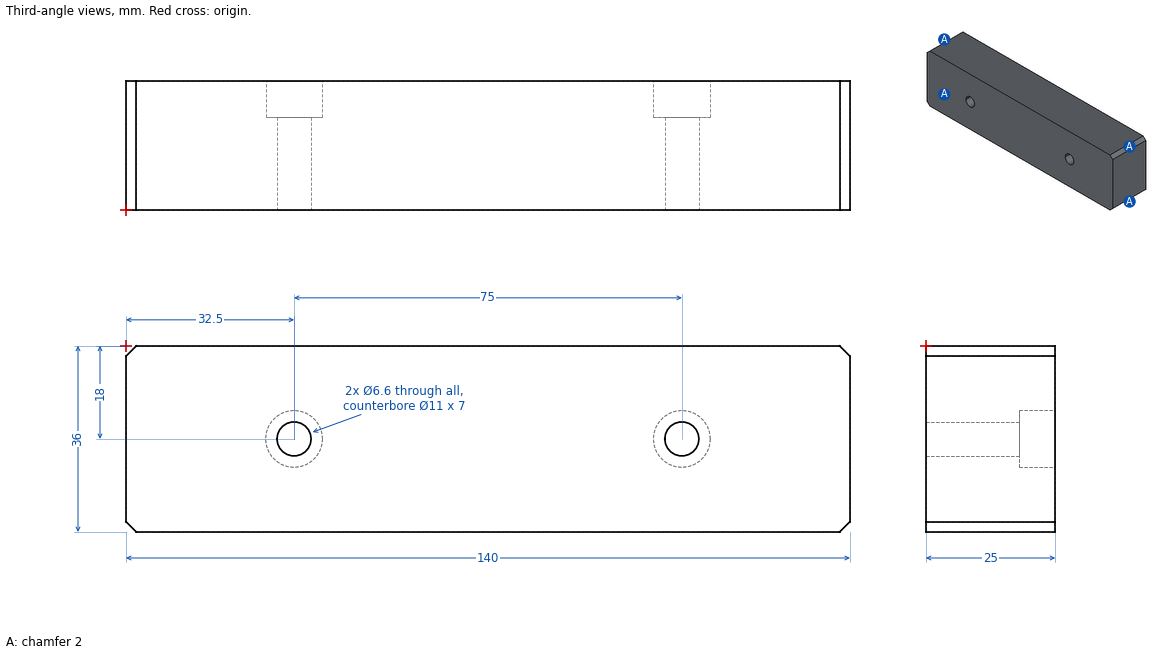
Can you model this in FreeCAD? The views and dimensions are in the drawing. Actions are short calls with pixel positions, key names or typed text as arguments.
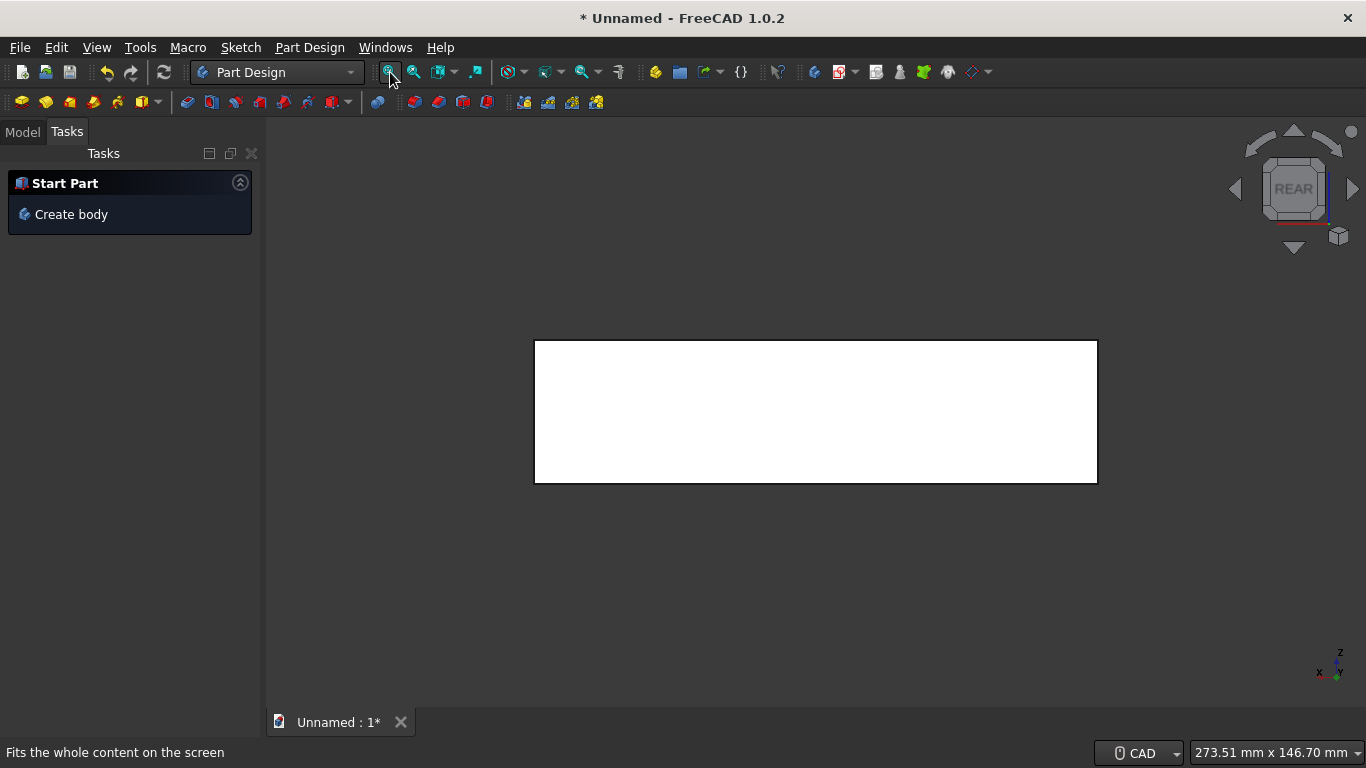
click(655, 411)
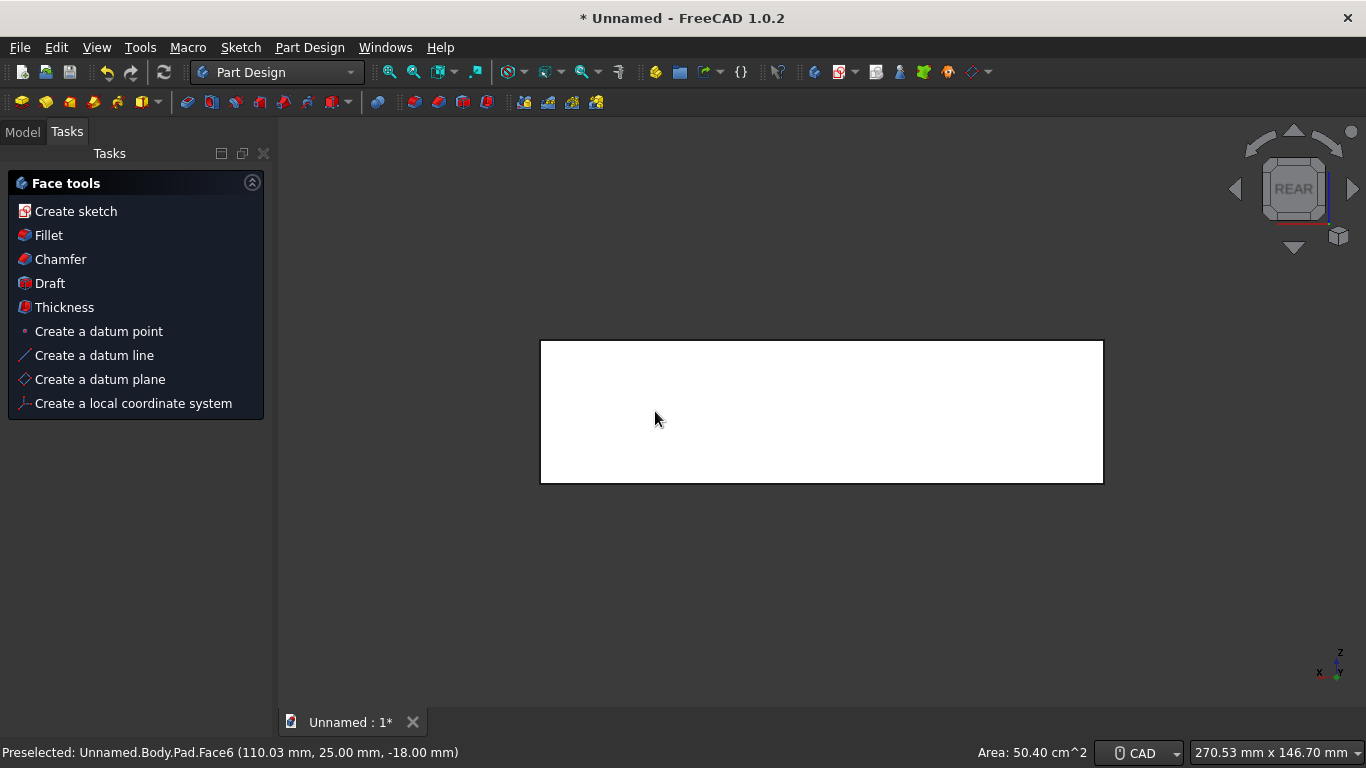
click(840, 72)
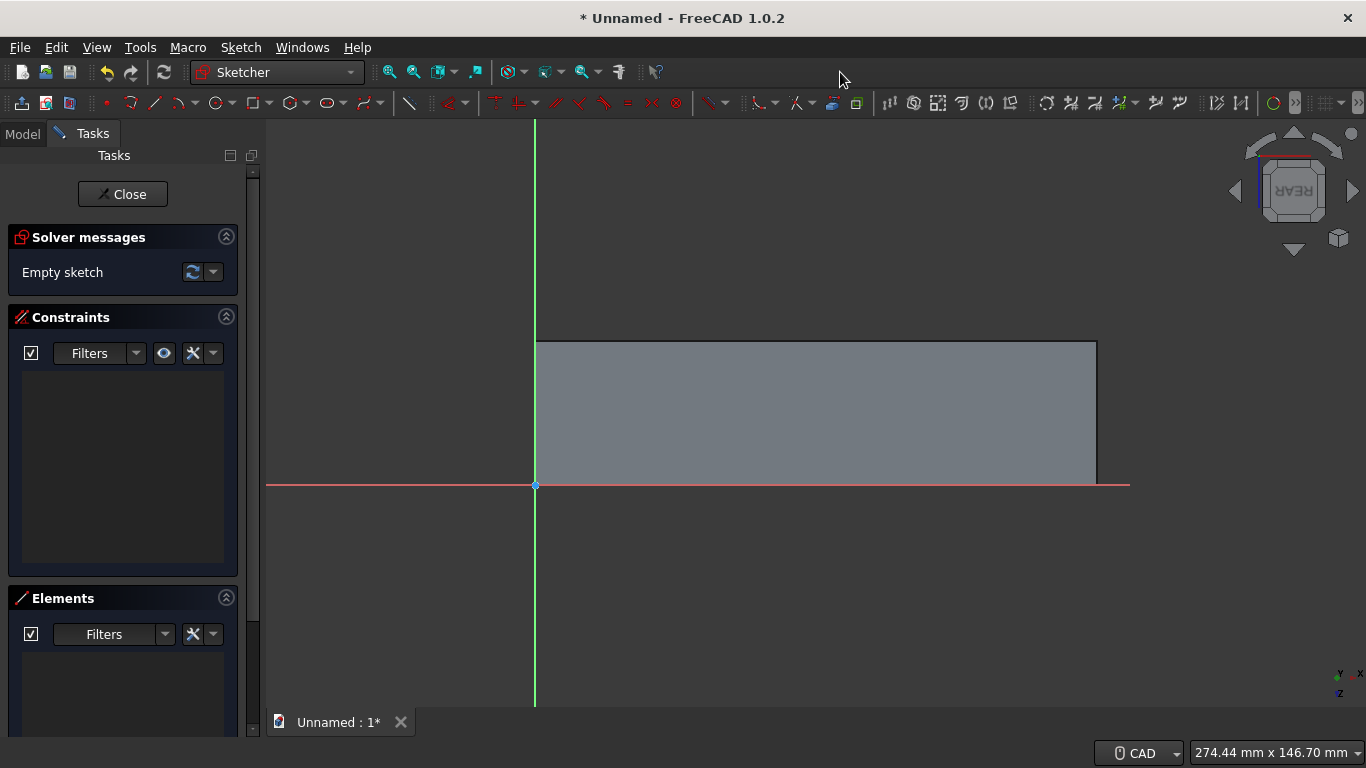
scroll(778, 502, up, 2)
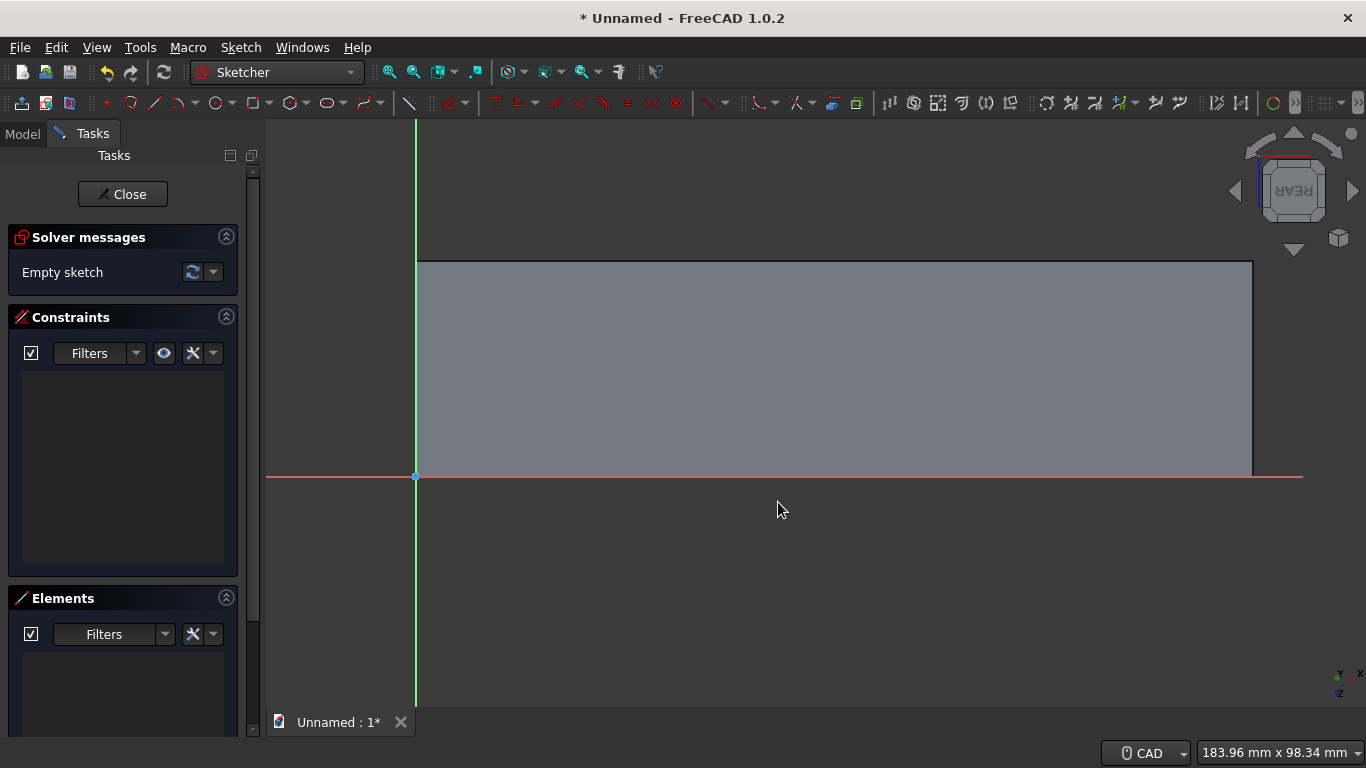
click(216, 104)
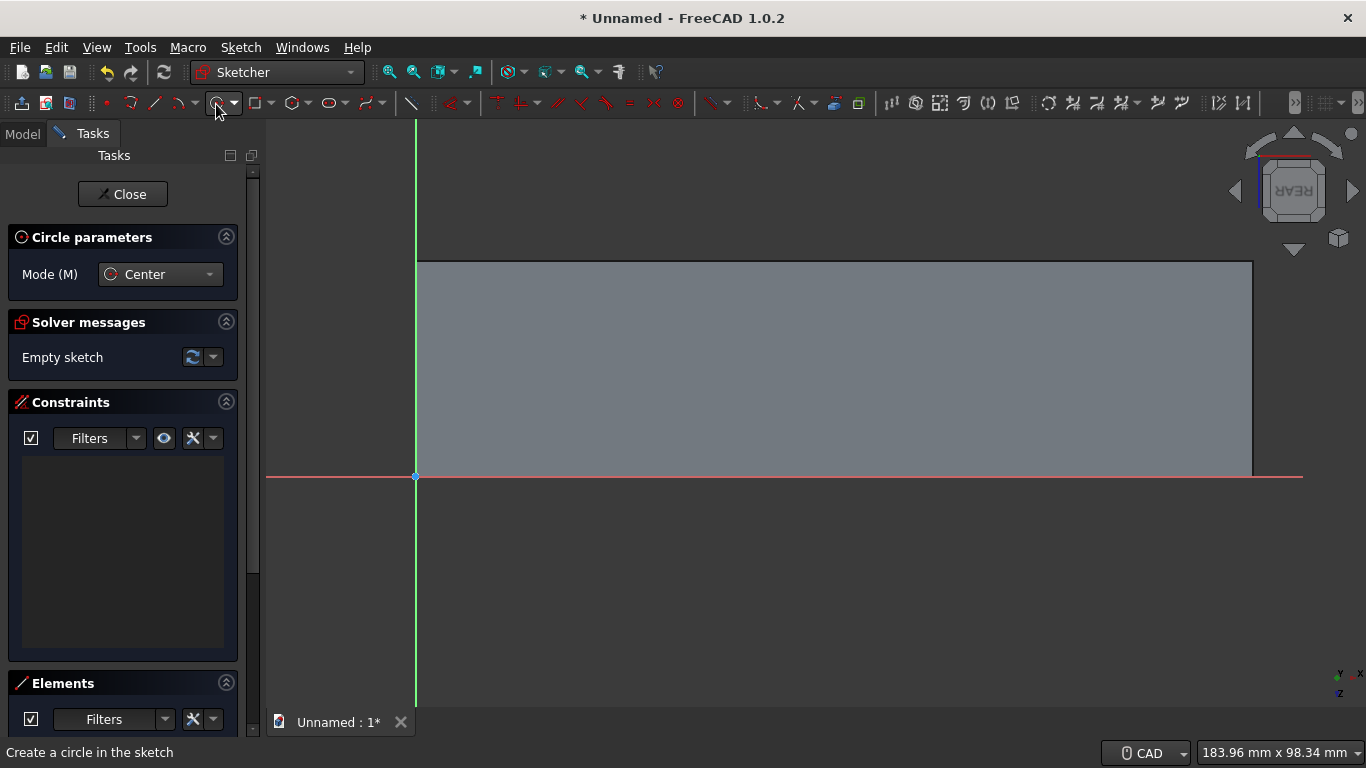
click(610, 369)
click(624, 355)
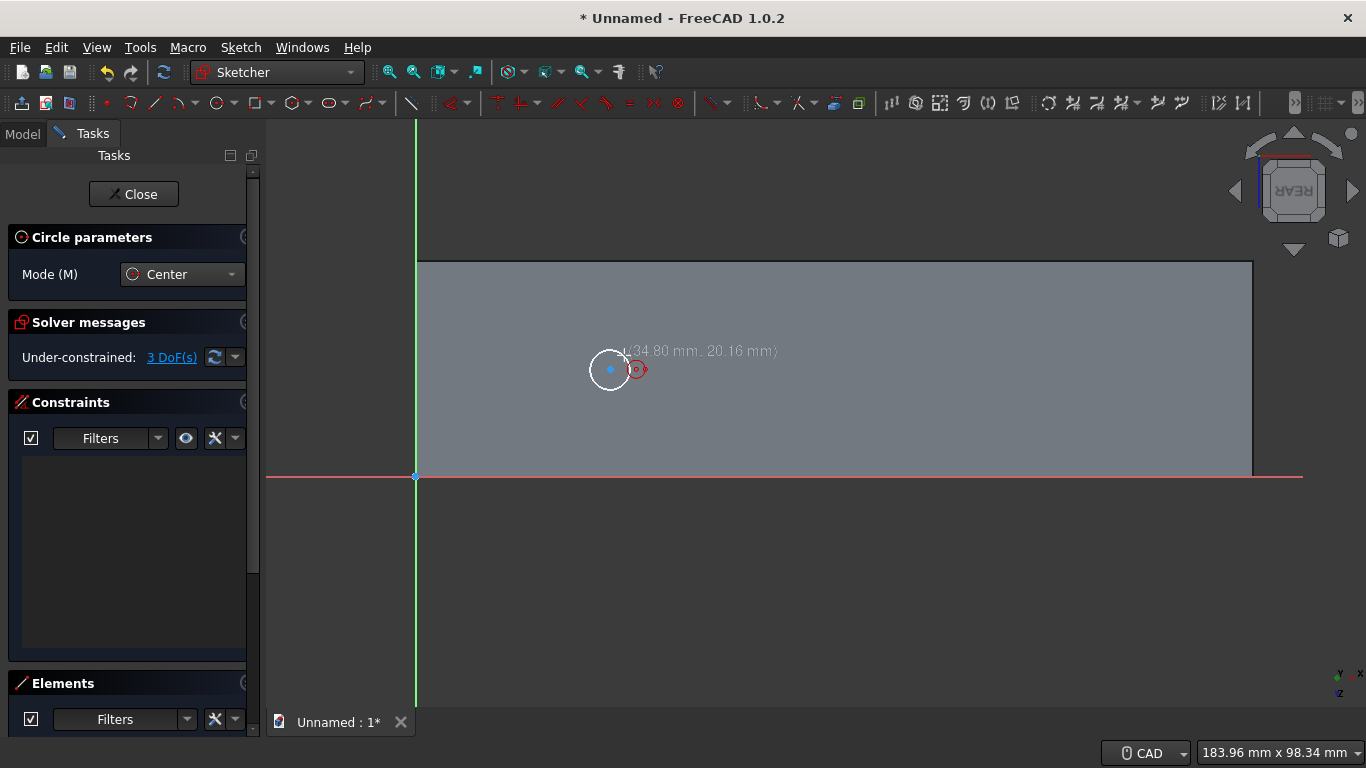
click(1059, 369)
click(1073, 355)
key(Escape)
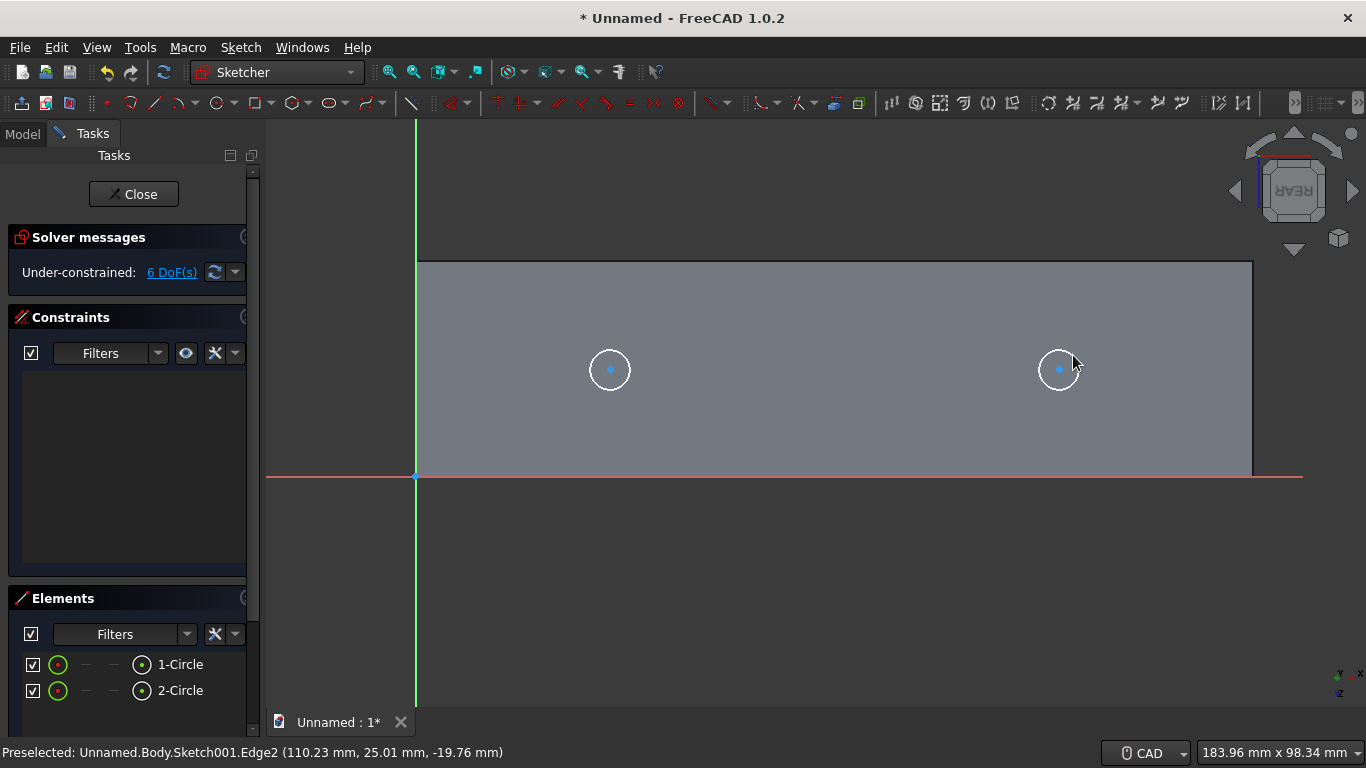
click(624, 356)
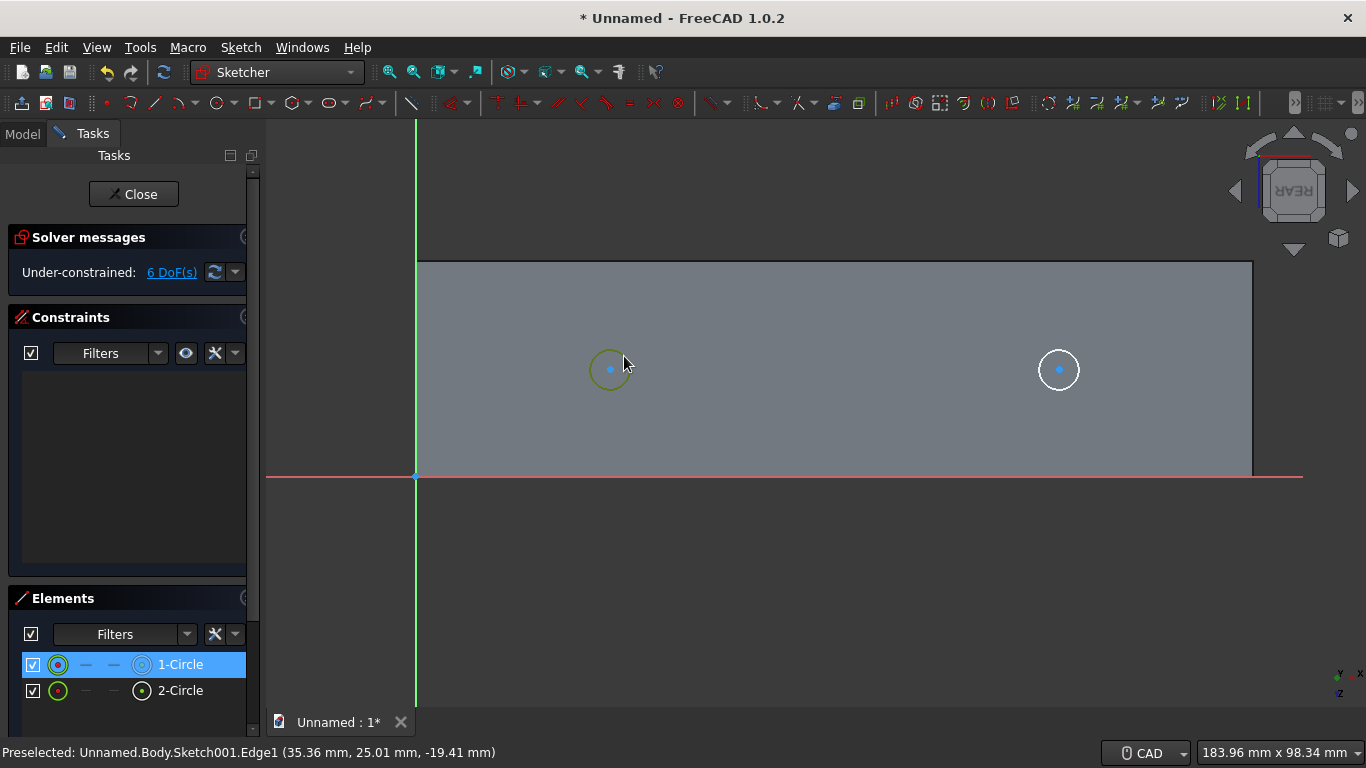
click(1073, 356)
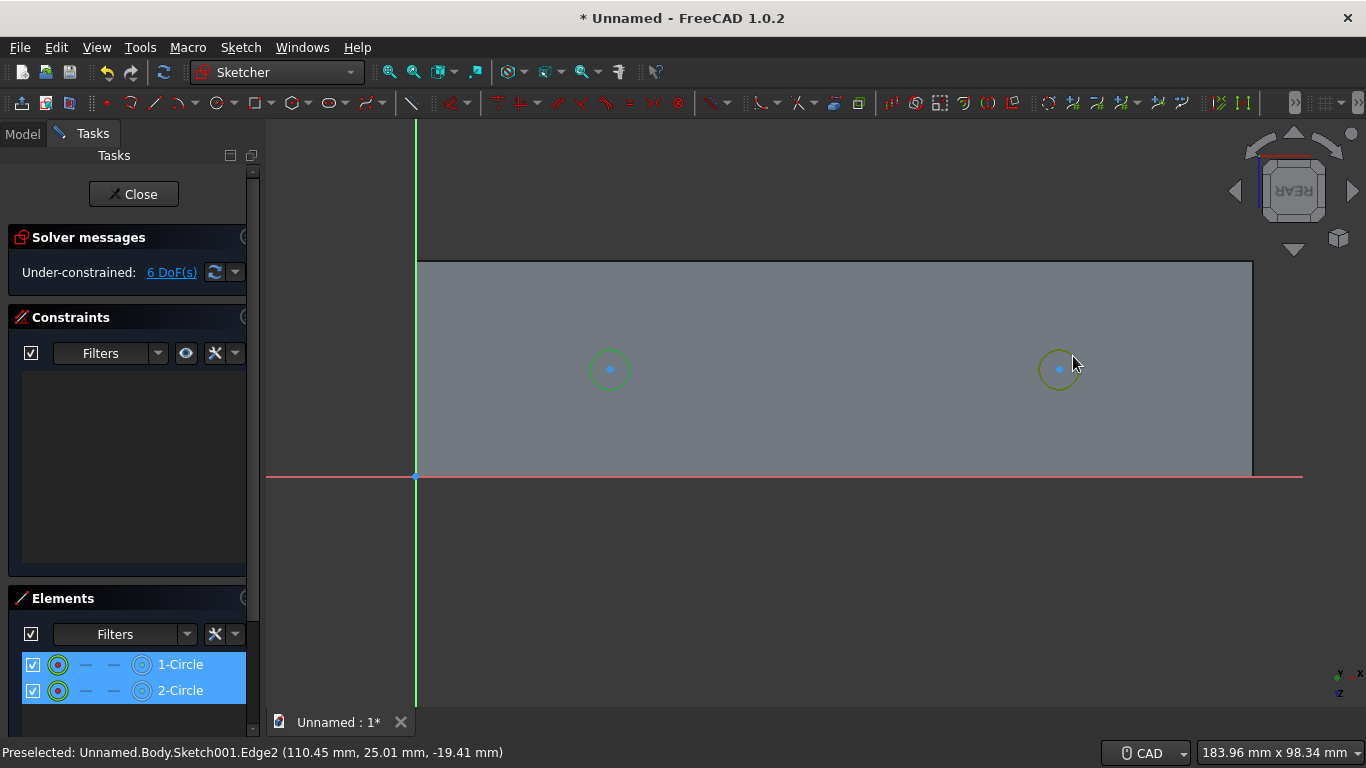
click(630, 104)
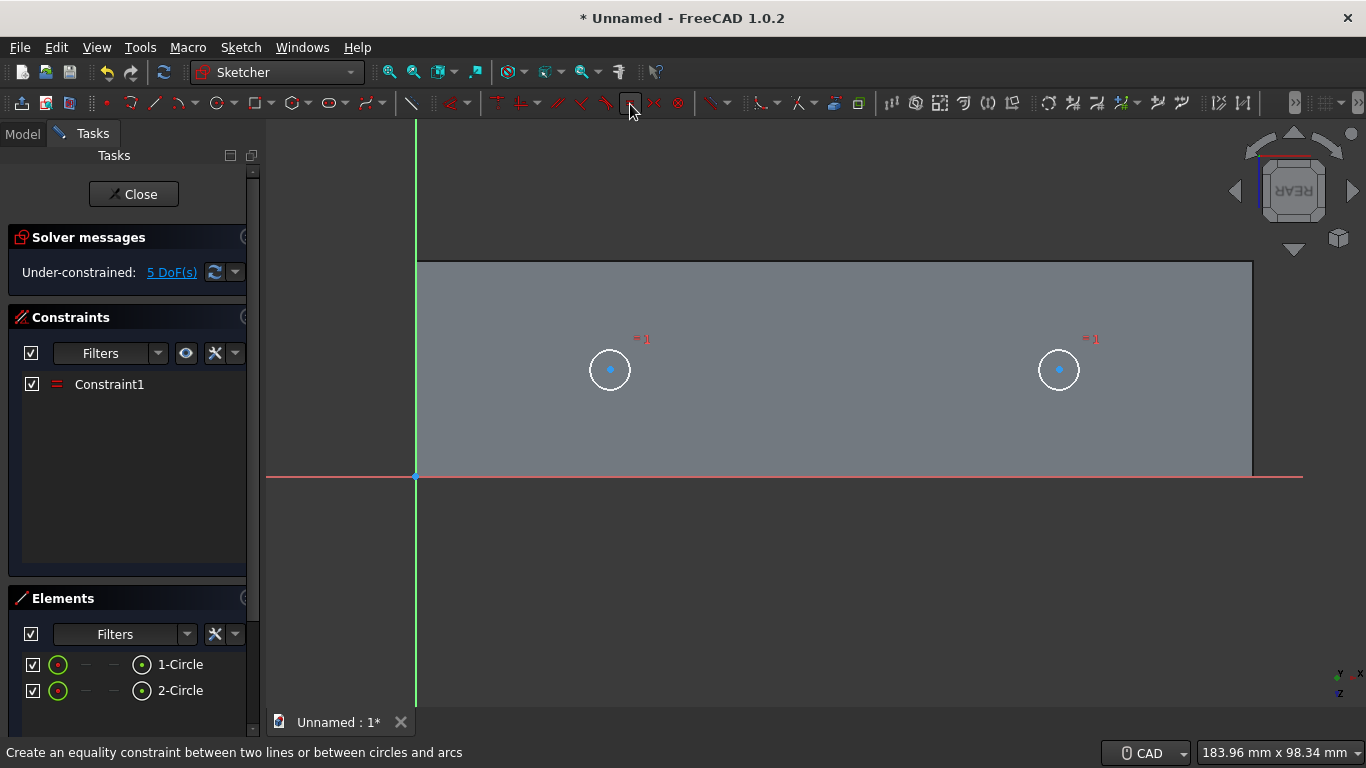
click(450, 104)